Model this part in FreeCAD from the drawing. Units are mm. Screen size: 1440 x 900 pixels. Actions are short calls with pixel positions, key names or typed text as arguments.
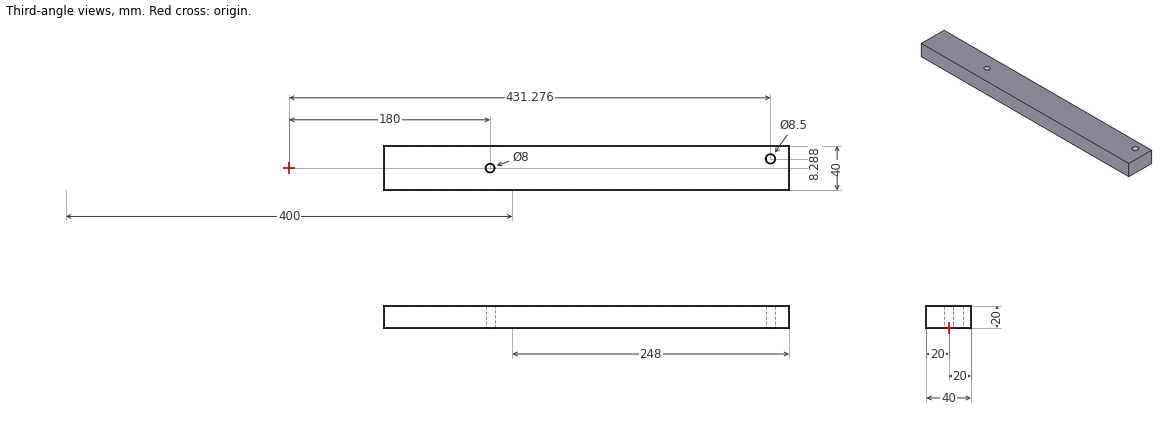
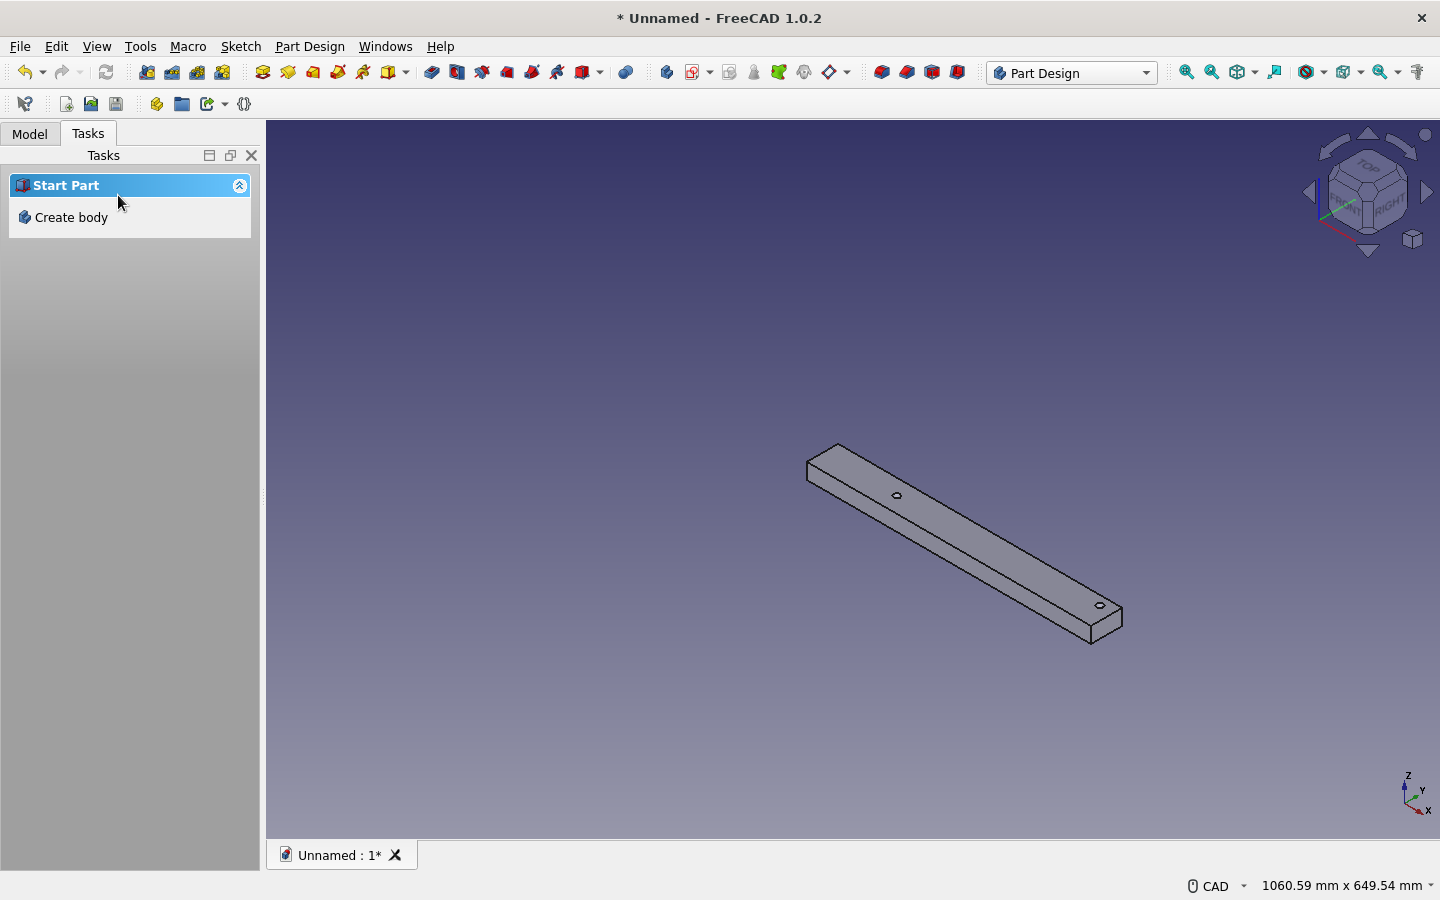
click(1187, 72)